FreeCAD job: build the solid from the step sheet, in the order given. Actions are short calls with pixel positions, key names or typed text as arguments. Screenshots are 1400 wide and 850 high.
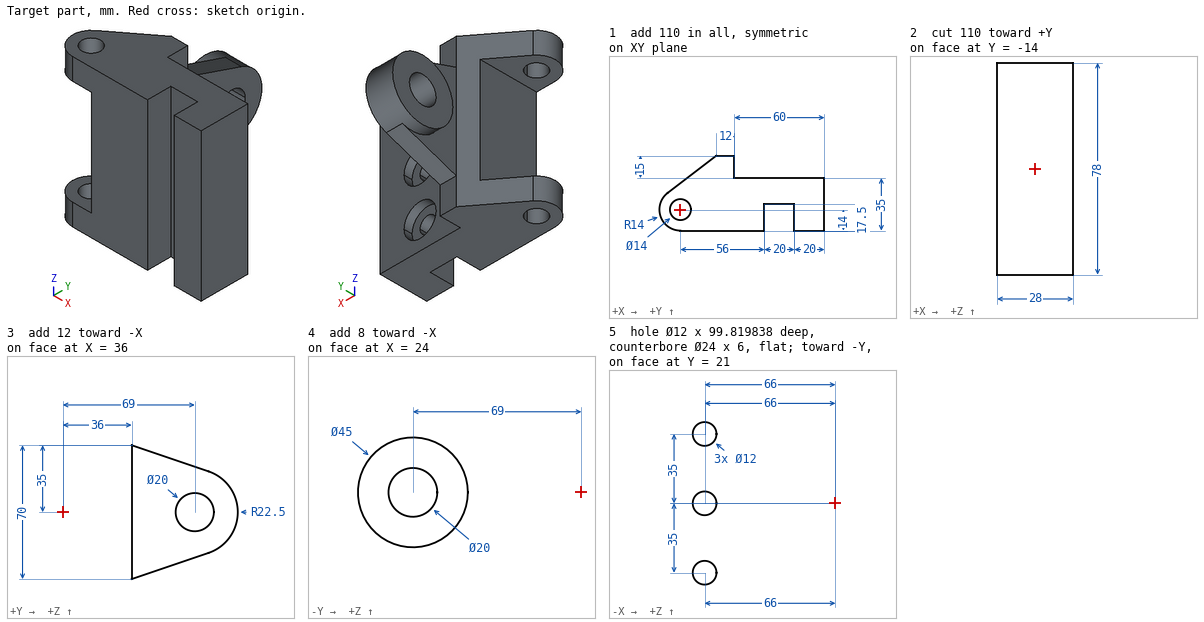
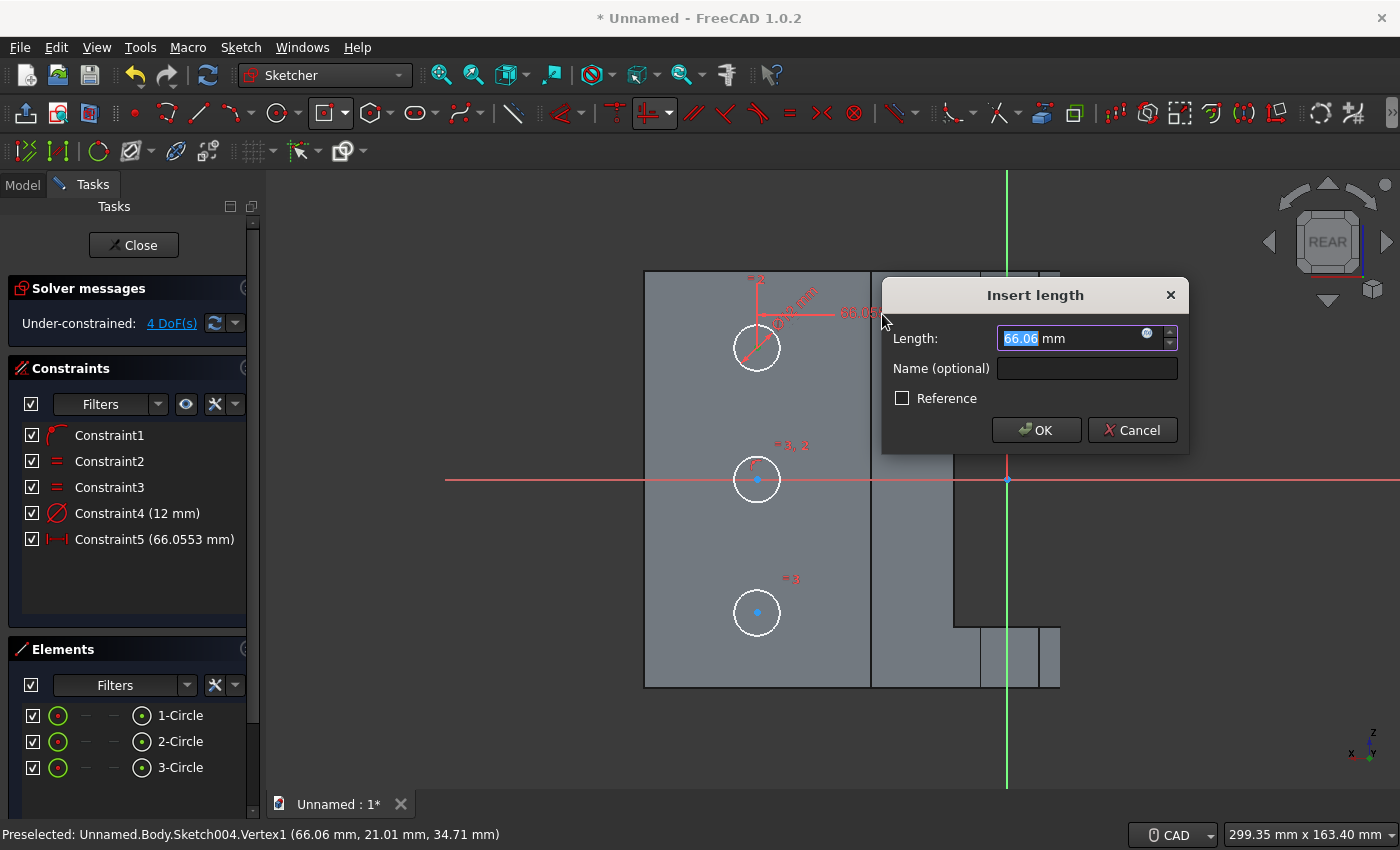
text(66)
key(Return)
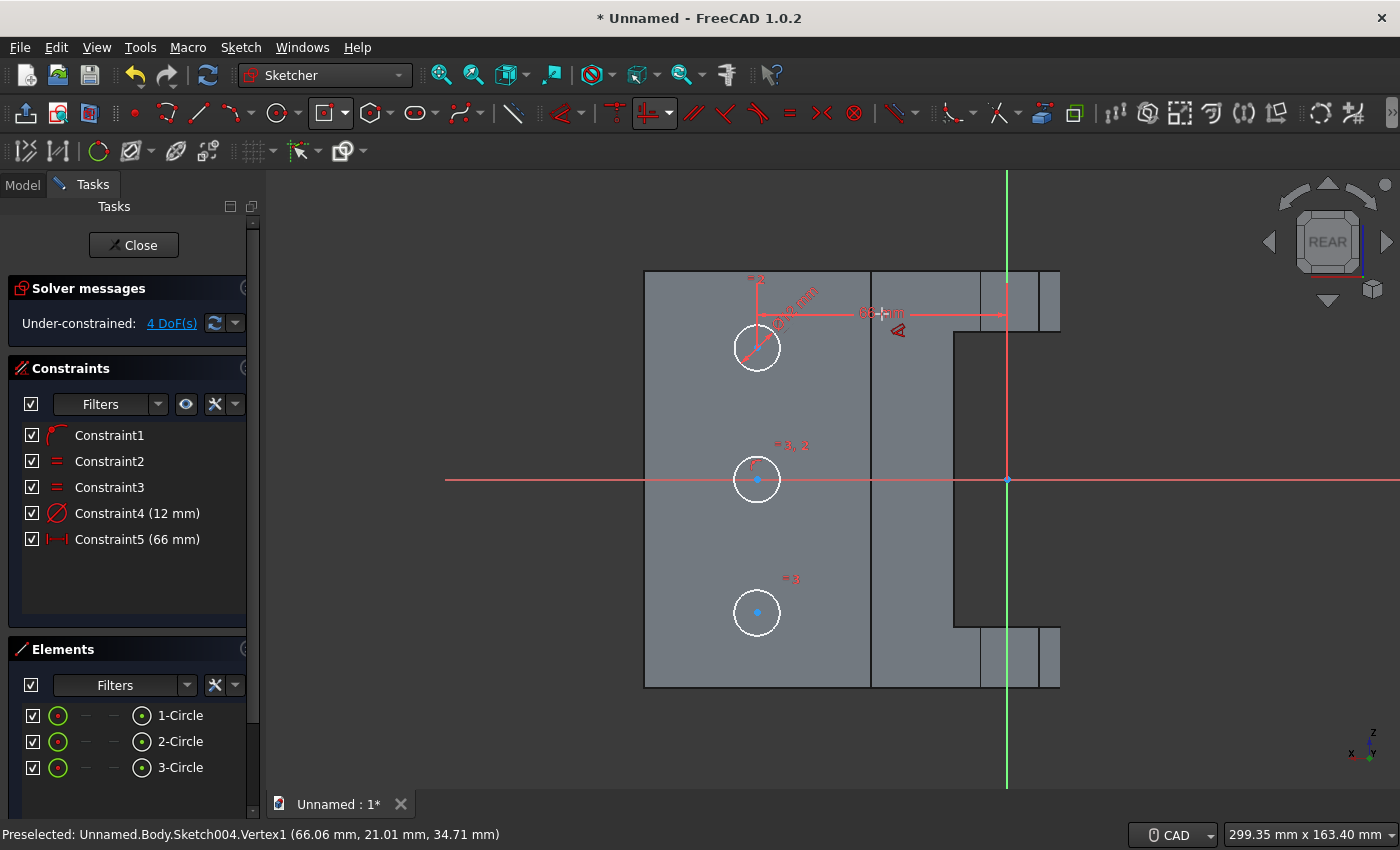
click(757, 348)
click(1041, 414)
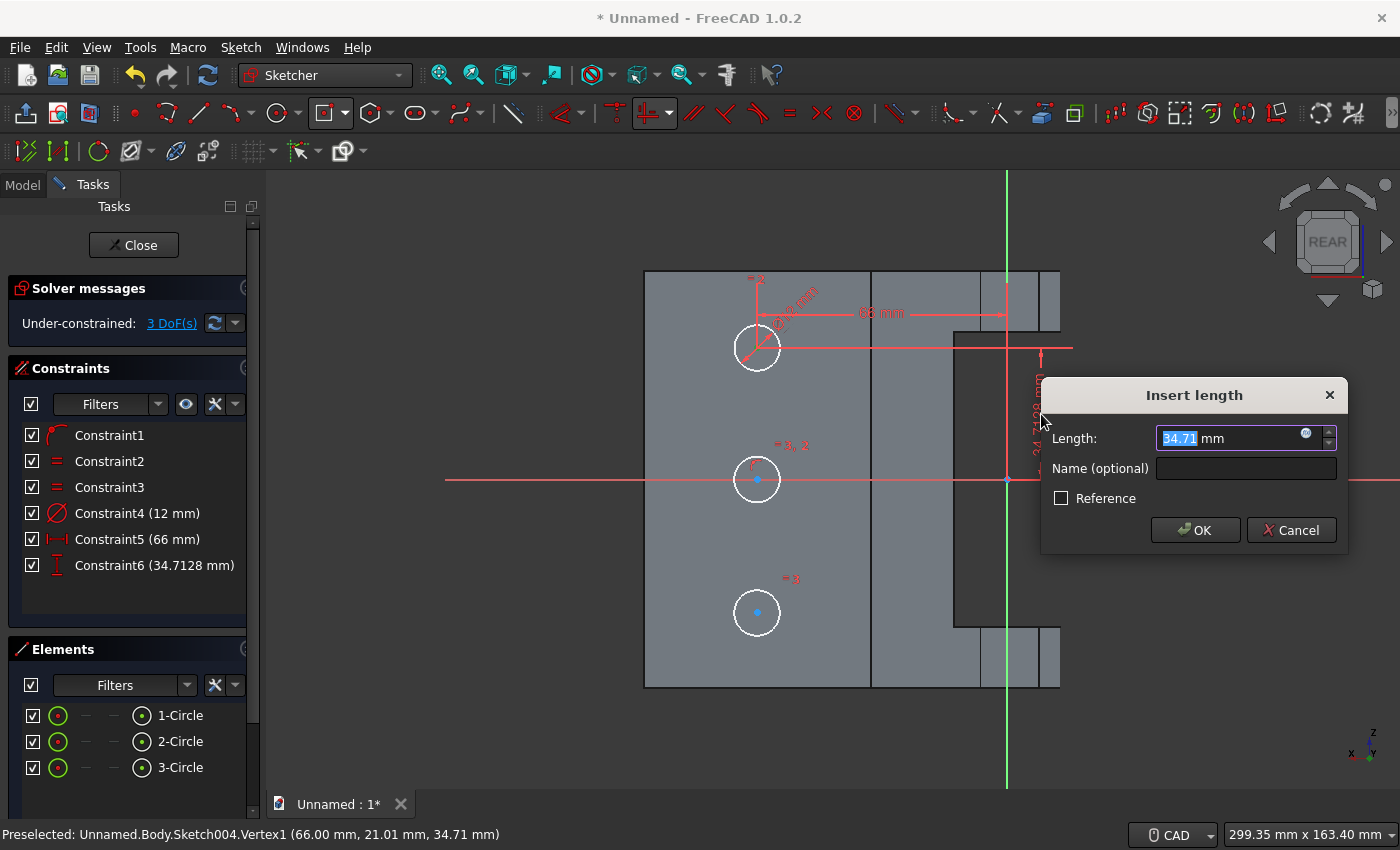
text(35)
key(Return)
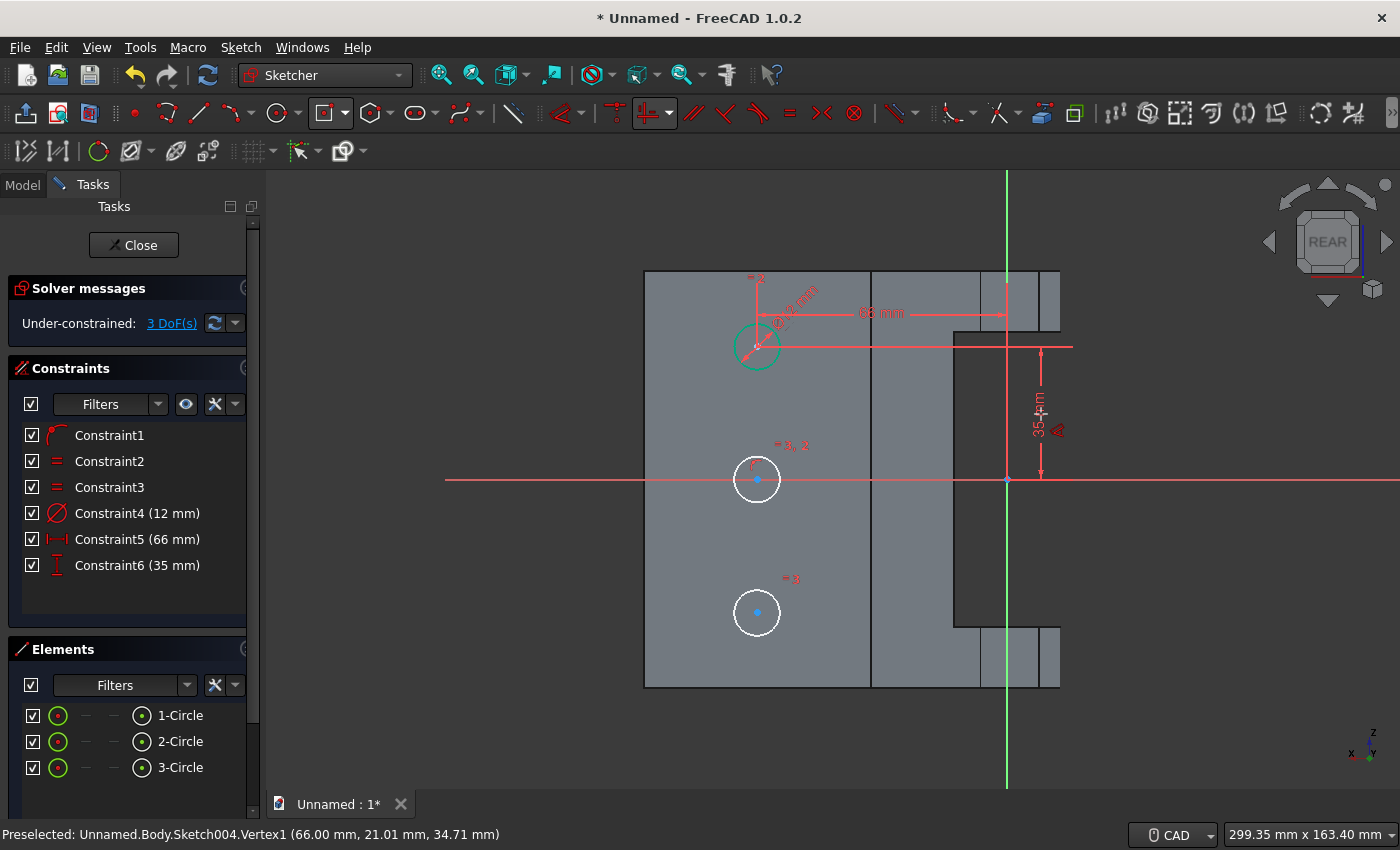
click(757, 480)
click(882, 514)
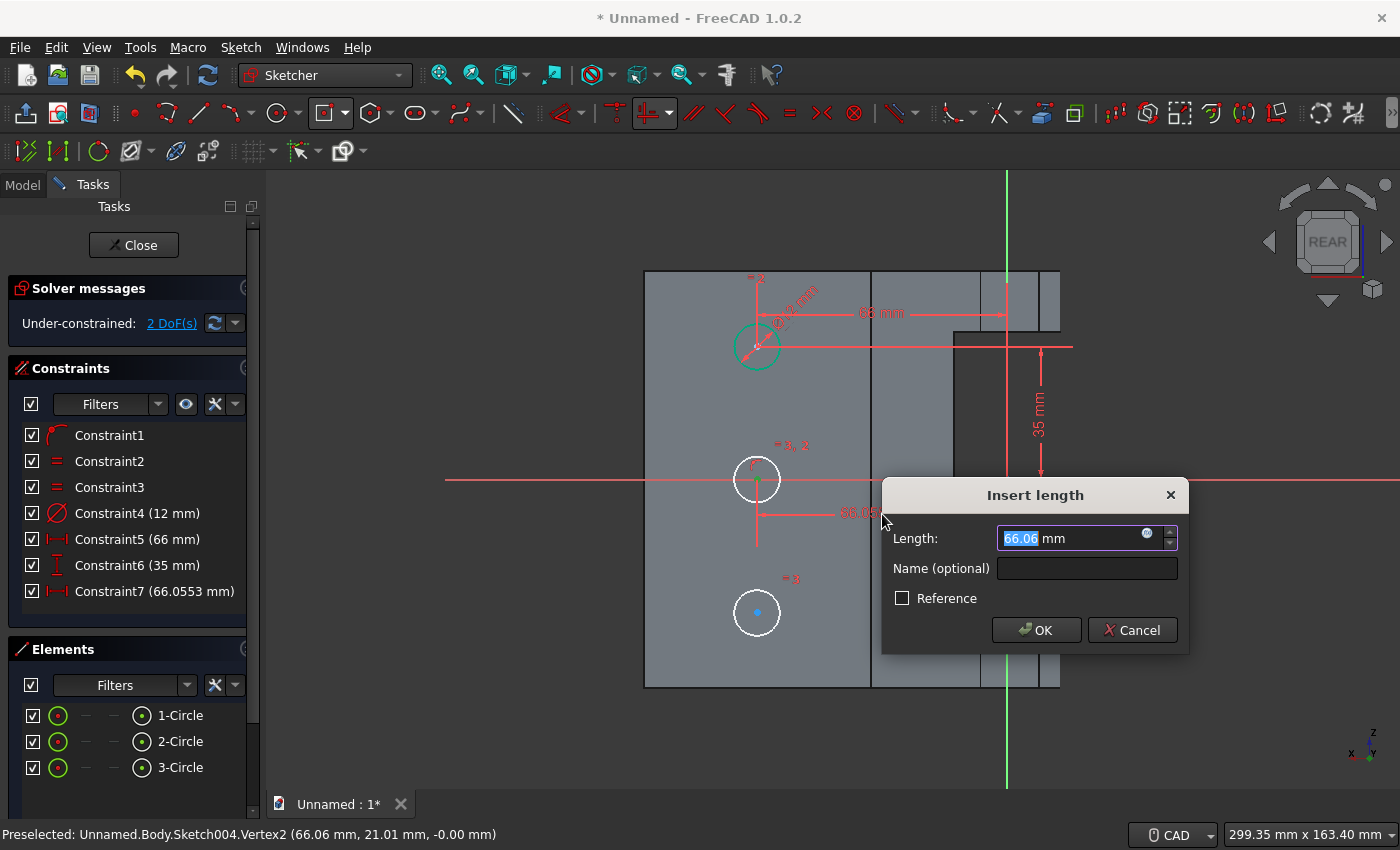
text(66)
key(Return)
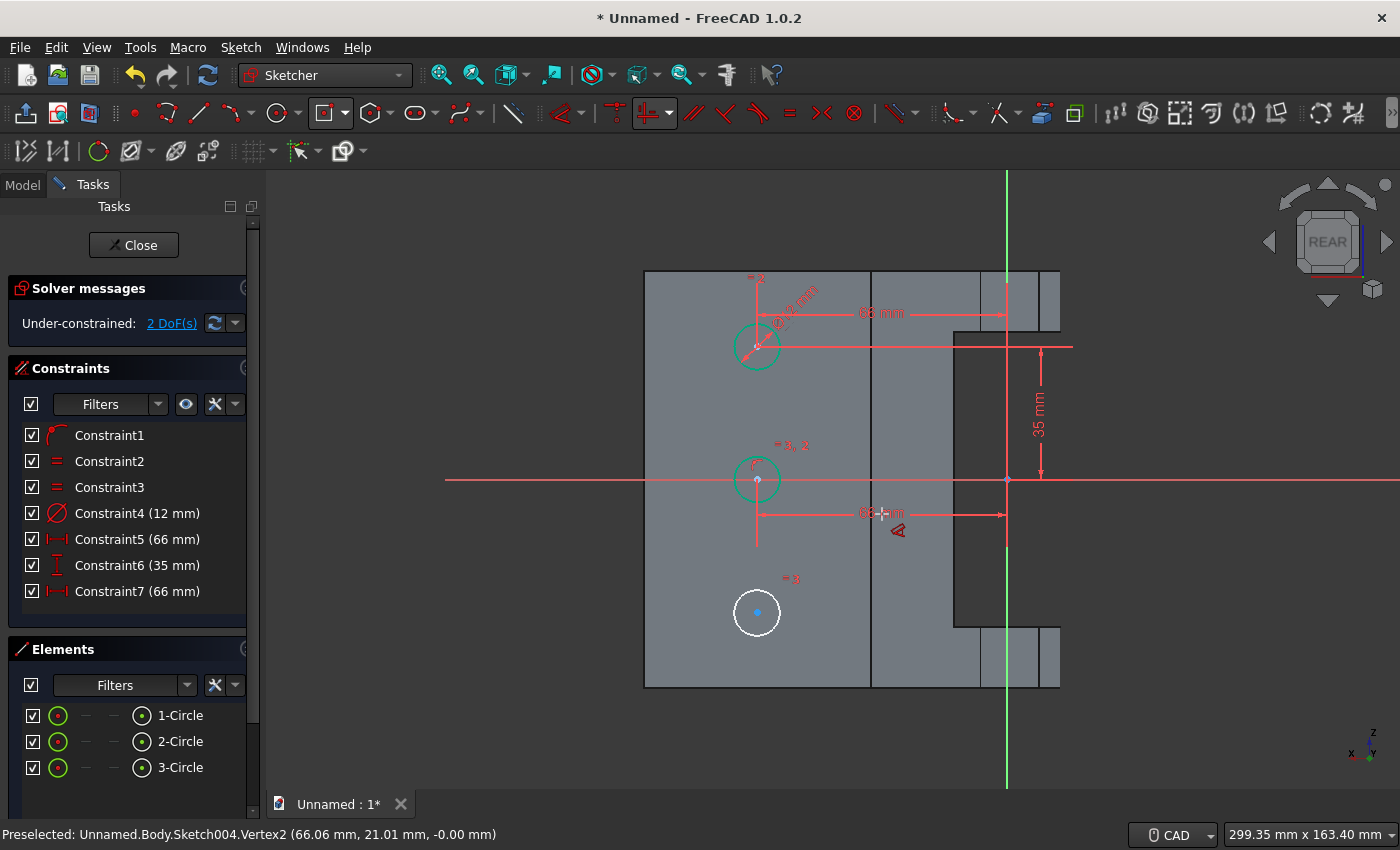
click(757, 613)
click(882, 647)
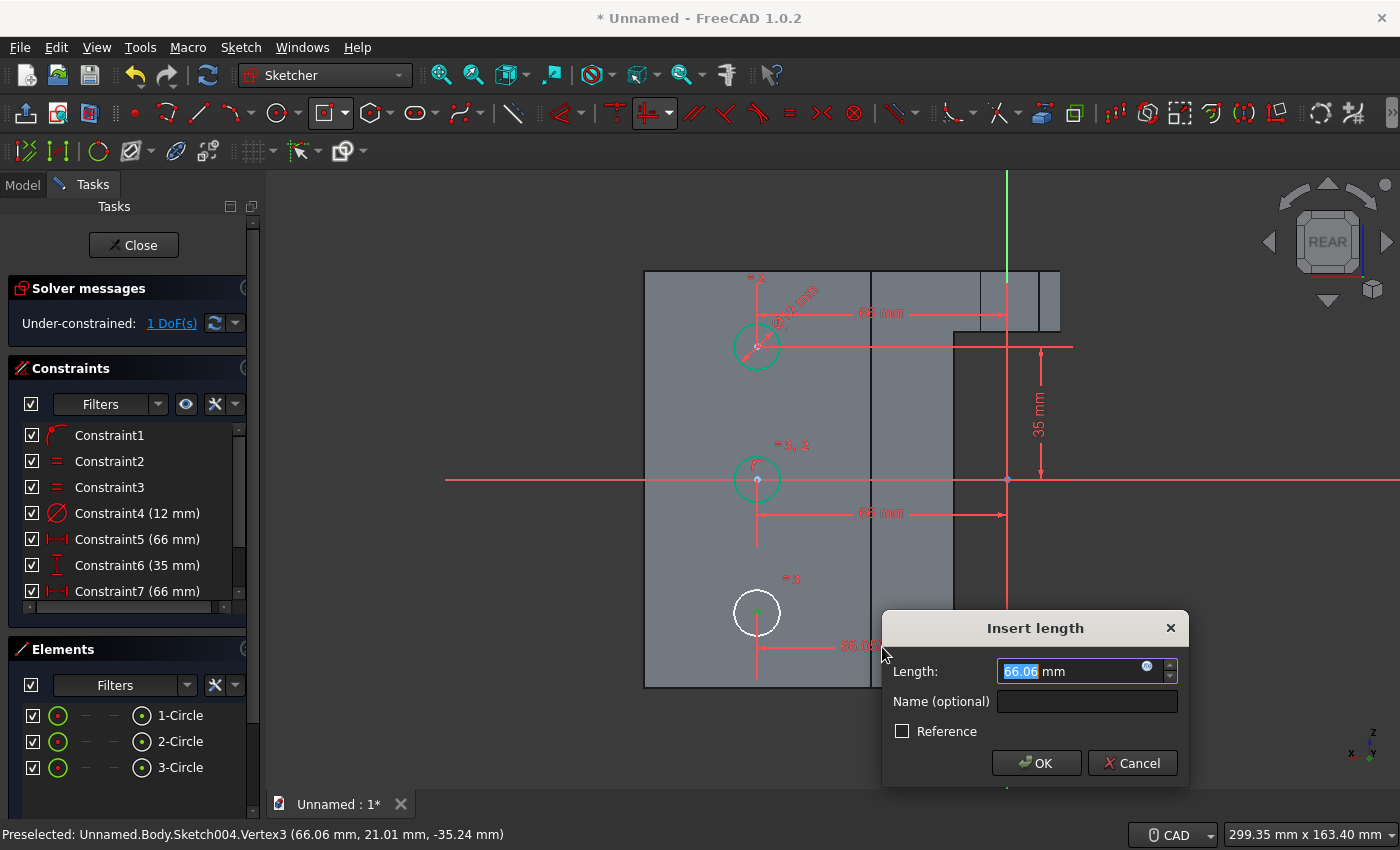
text(66)
key(Return)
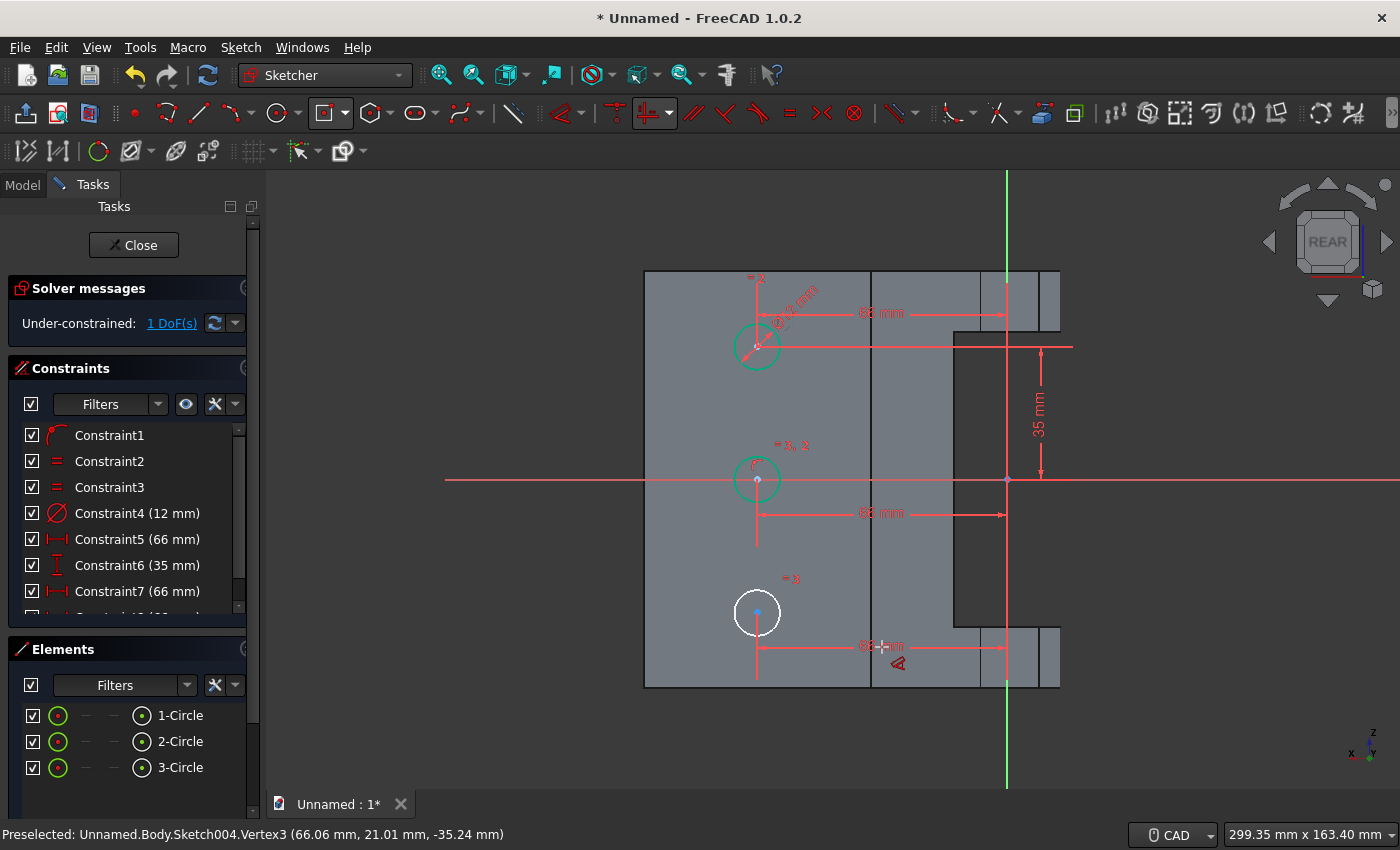
click(757, 613)
click(1041, 546)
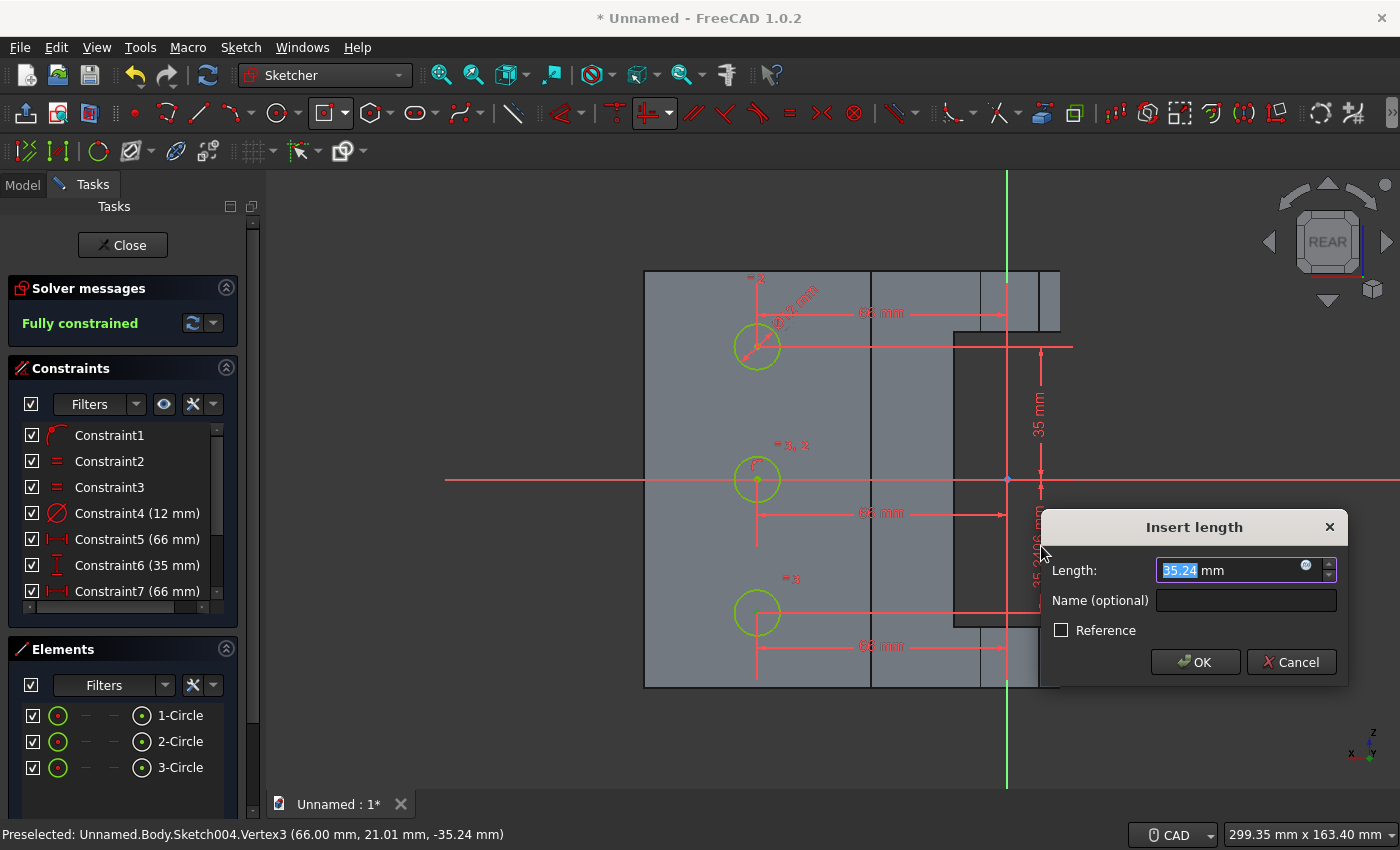
text(35)
key(Return)
key(Escape)